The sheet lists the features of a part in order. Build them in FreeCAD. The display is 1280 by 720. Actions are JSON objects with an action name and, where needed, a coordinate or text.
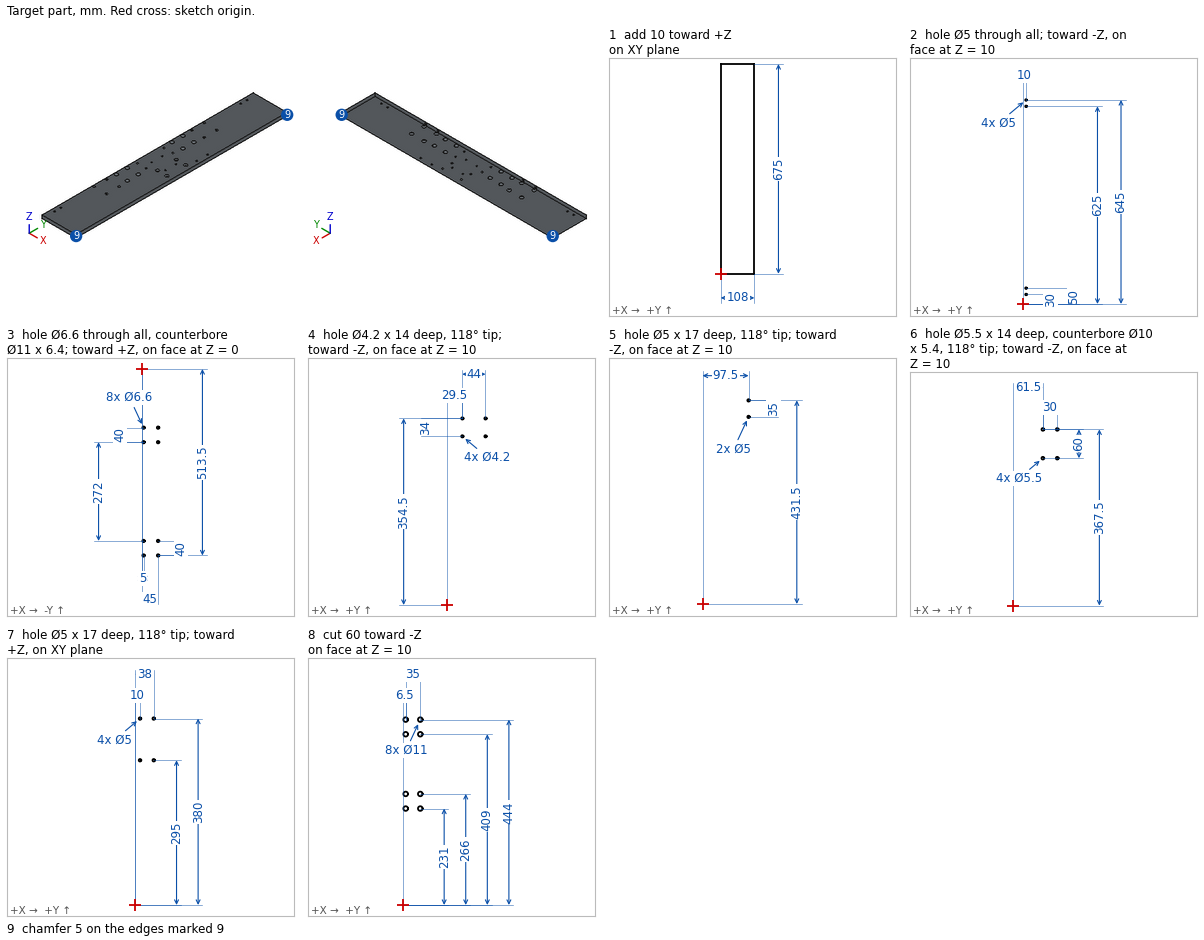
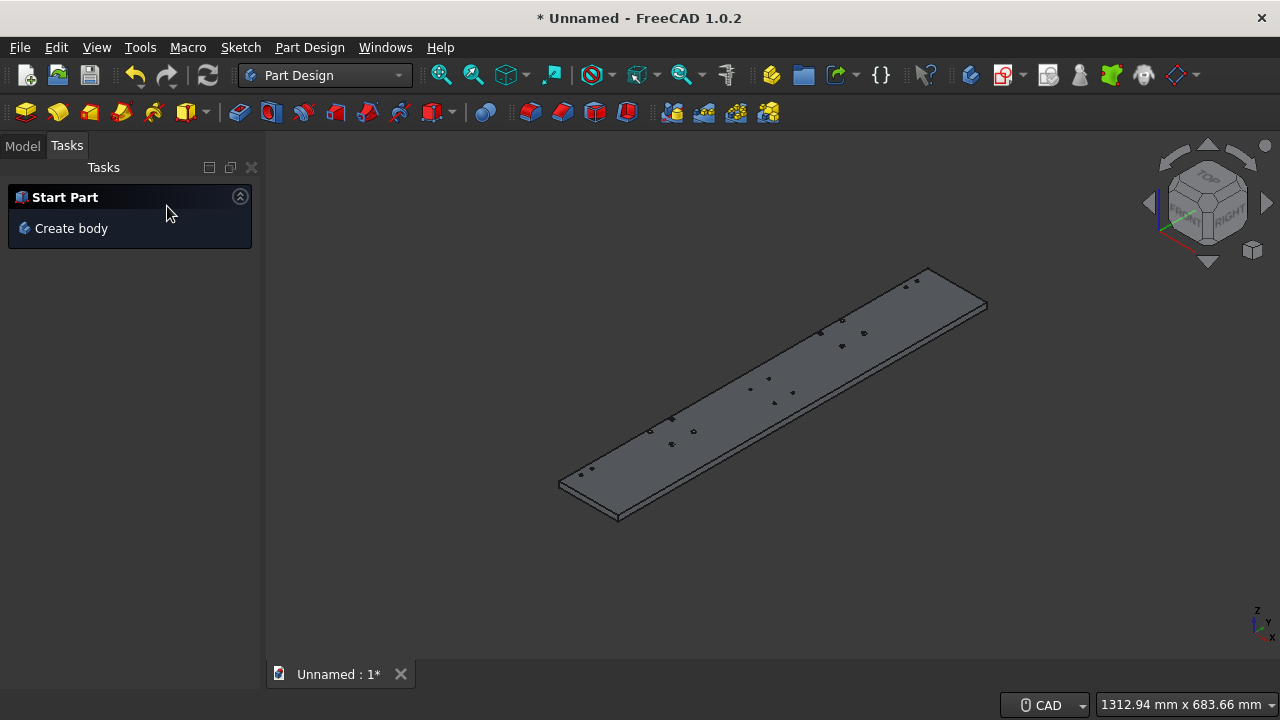
{"action": "left_click", "coordinate": [931, 300]}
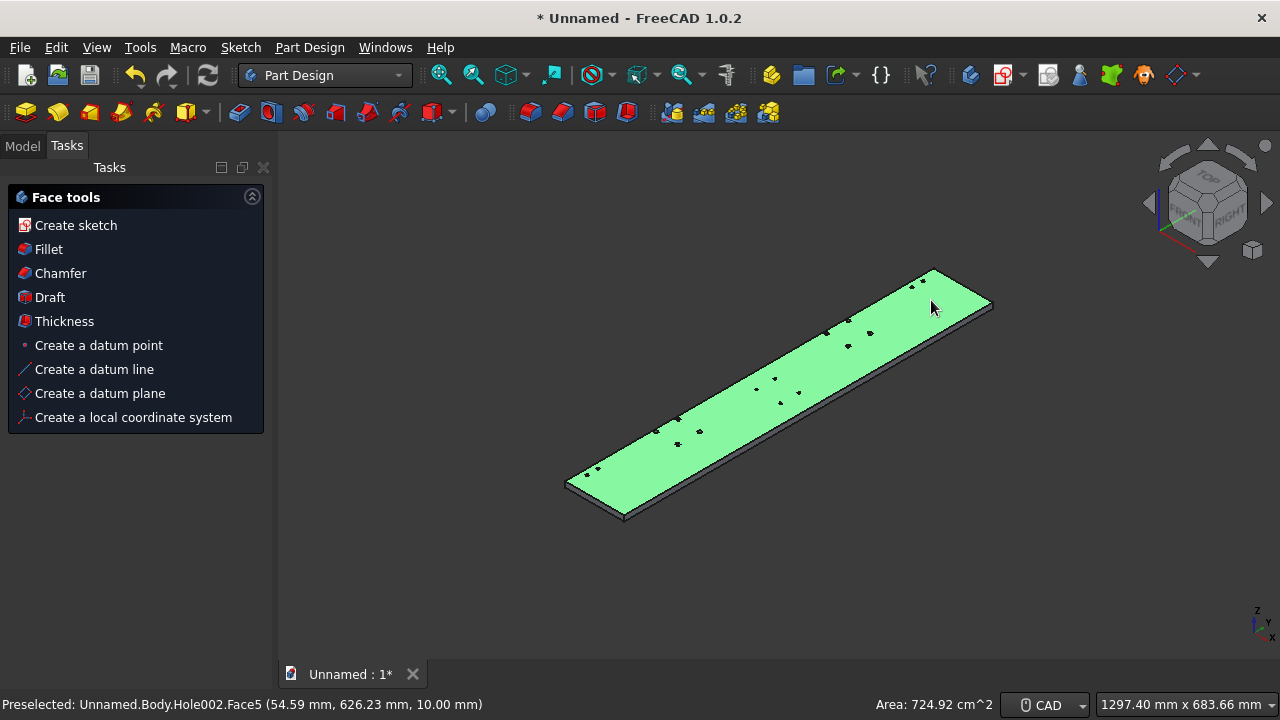
{"action": "left_click", "coordinate": [1004, 76]}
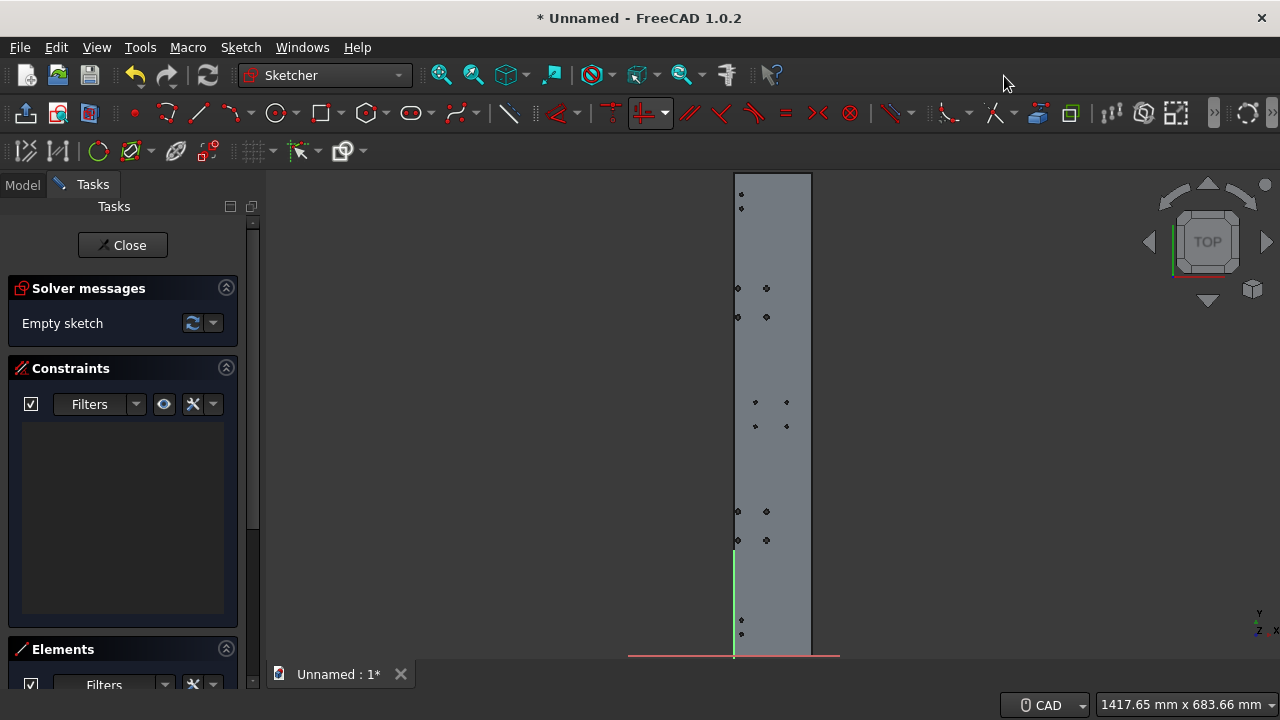
{"action": "scroll", "coordinate": [814, 354], "scroll_direction": "up", "scroll_amount": 12}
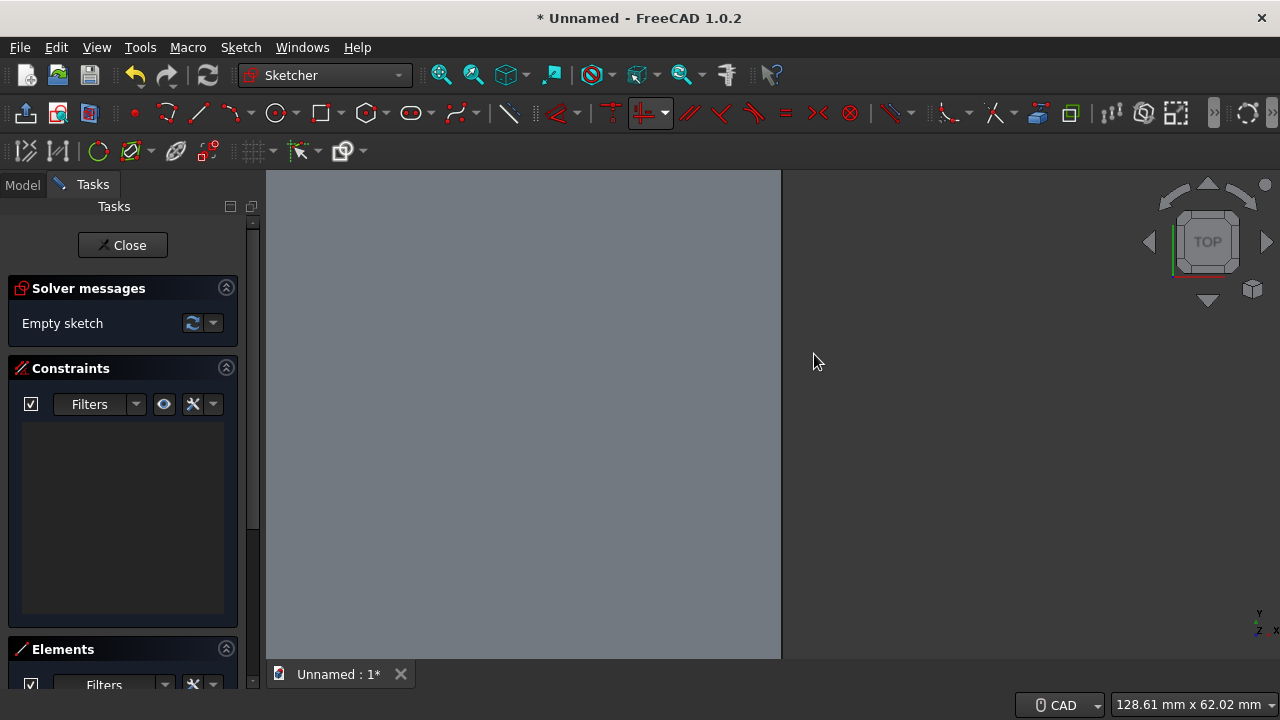
{"action": "left_click", "coordinate": [276, 114]}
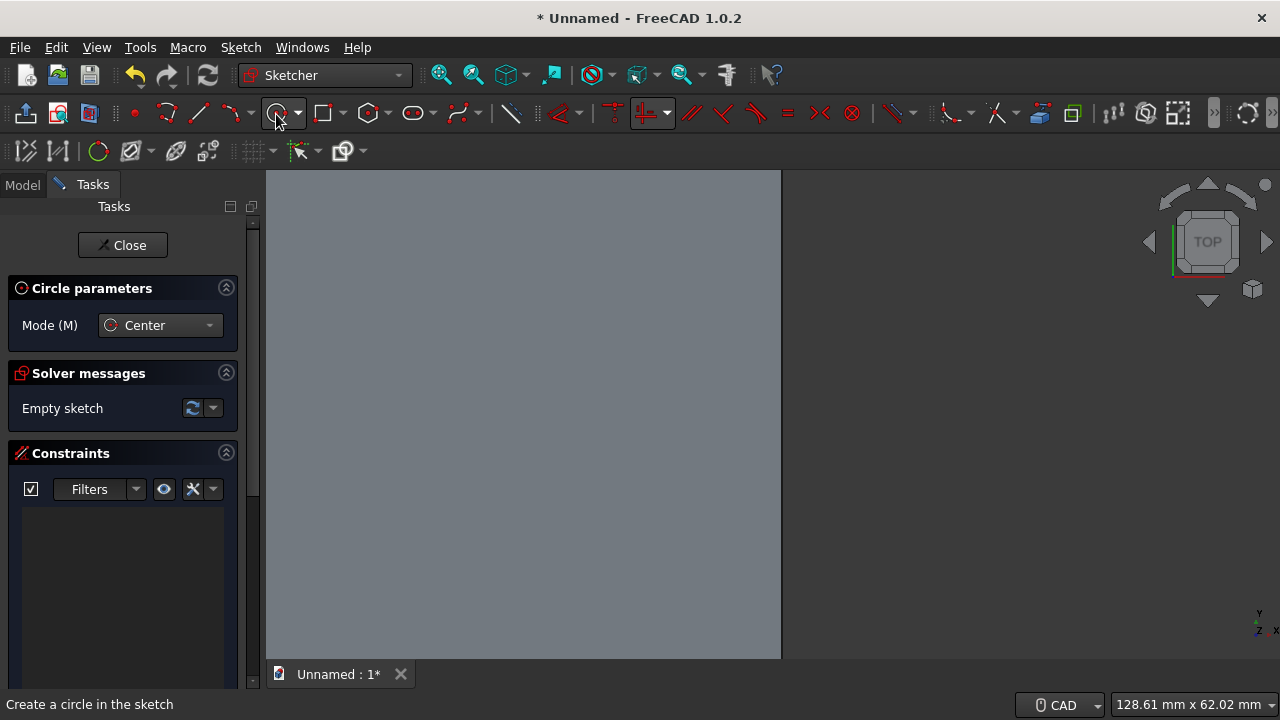
{"action": "left_click", "coordinate": [700, 276]}
{"action": "mouse_move", "coordinate": [714, 262]}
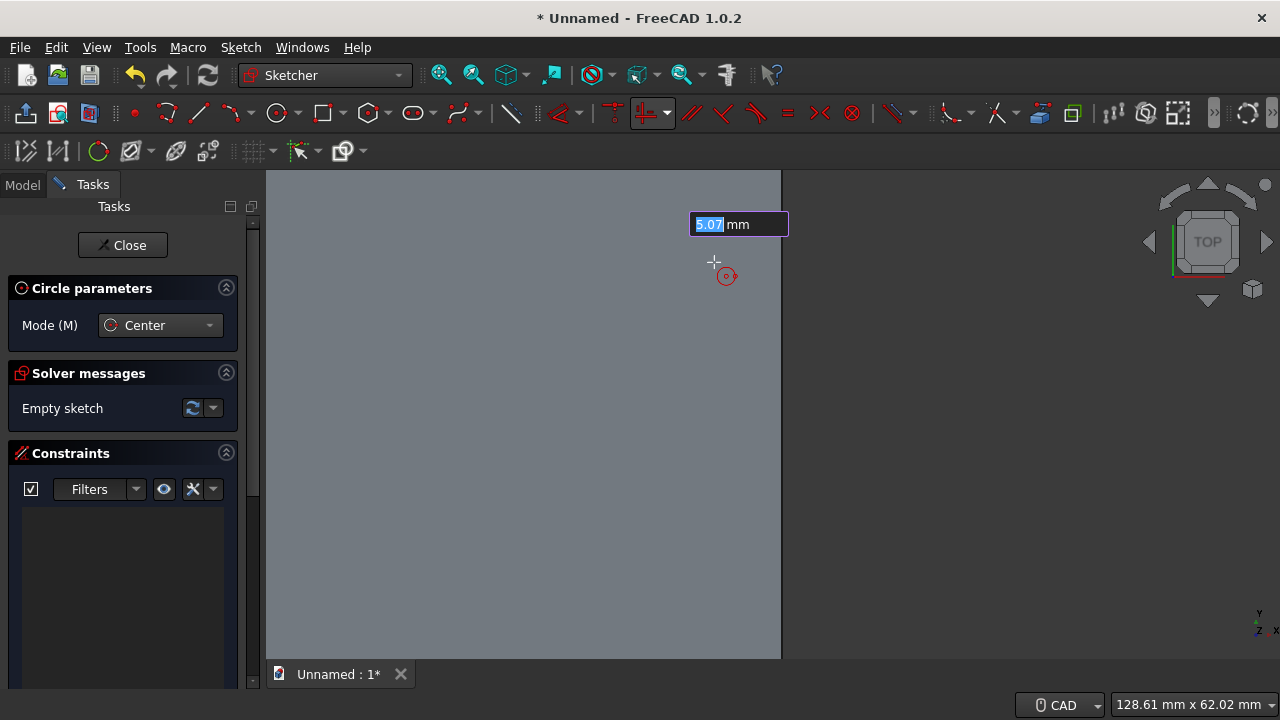
{"action": "type", "text": "5"}
{"action": "key", "text": "Return"}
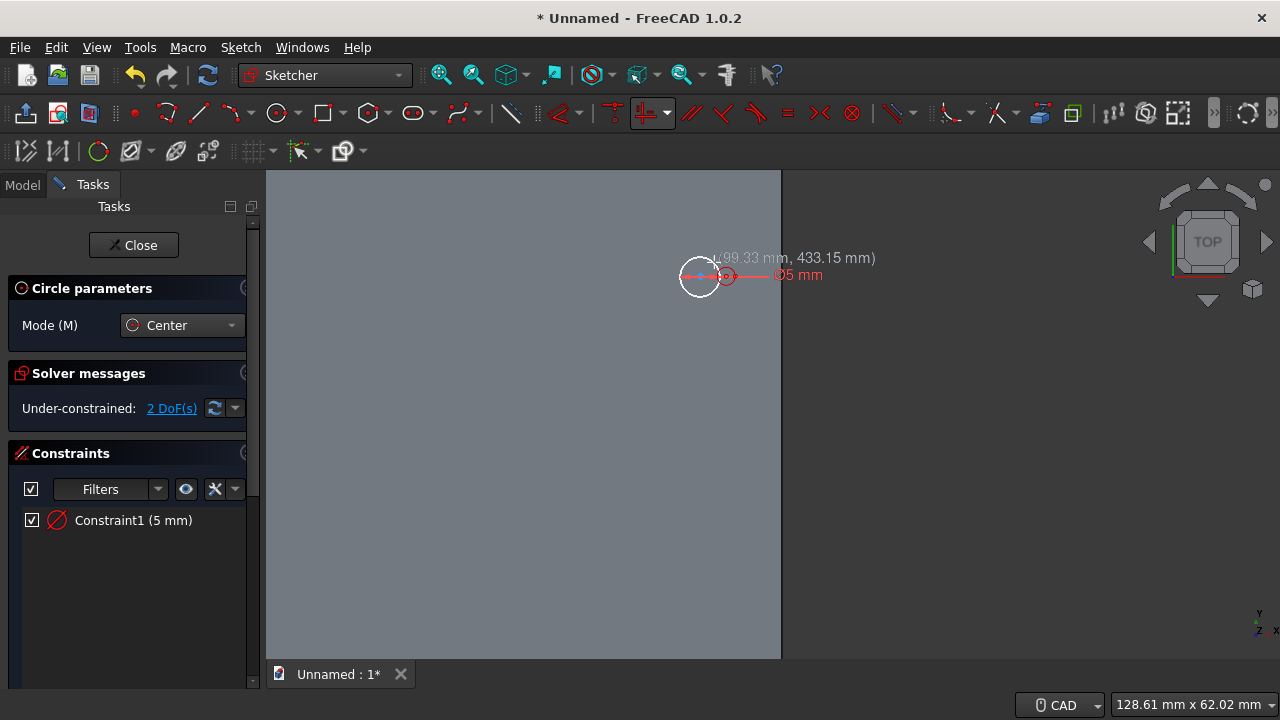
{"action": "left_click", "coordinate": [700, 552]}
{"action": "mouse_move", "coordinate": [714, 538]}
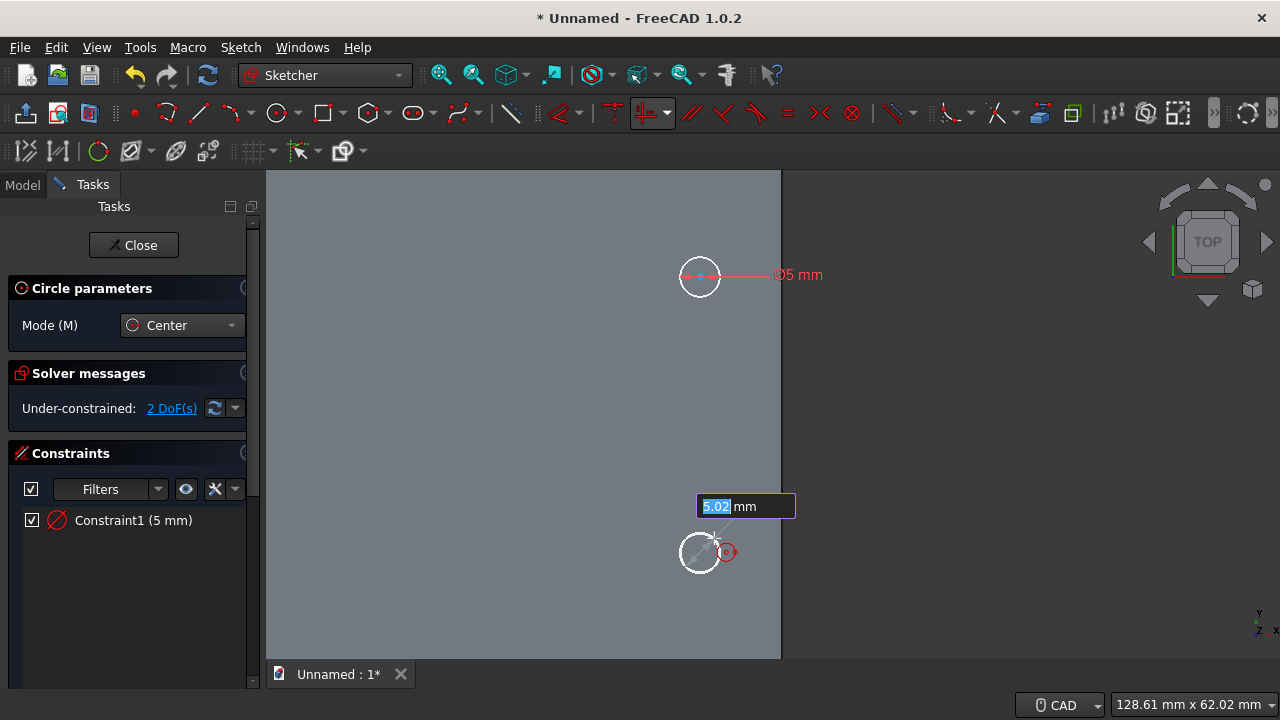
{"action": "type", "text": "5"}
{"action": "key", "text": "Return"}
{"action": "key", "text": "Escape"}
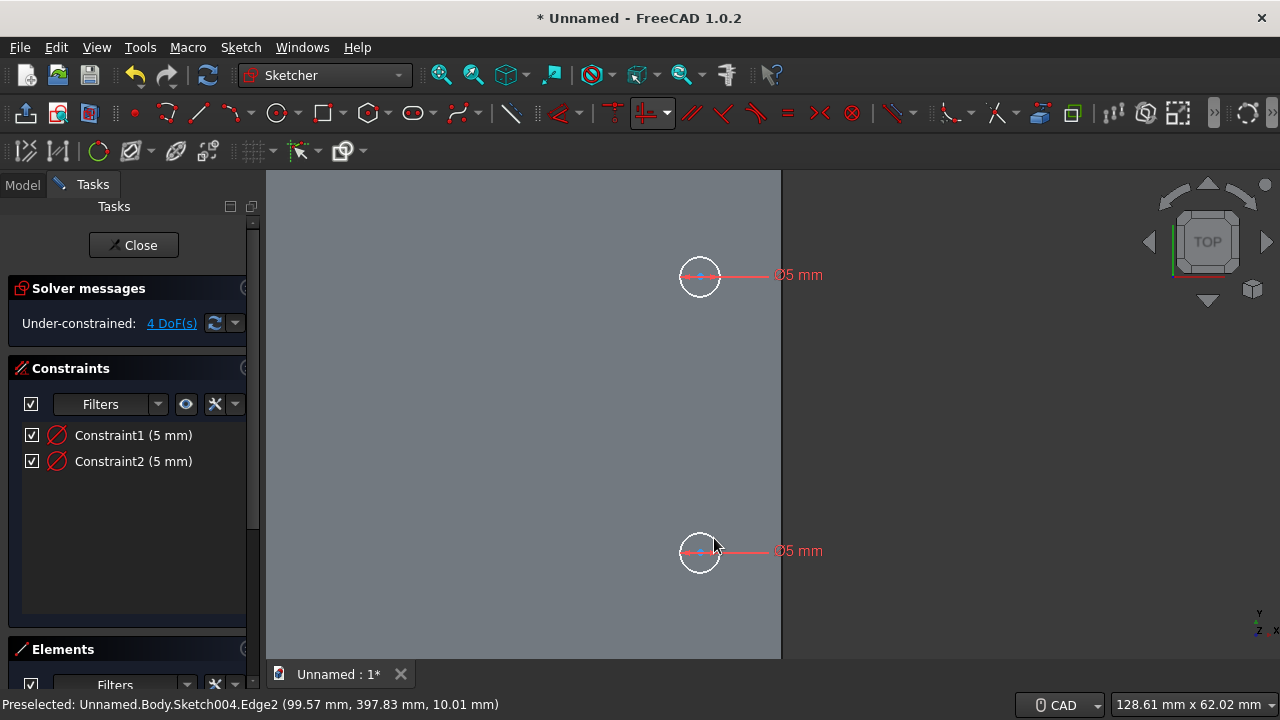
{"action": "left_click", "coordinate": [700, 277]}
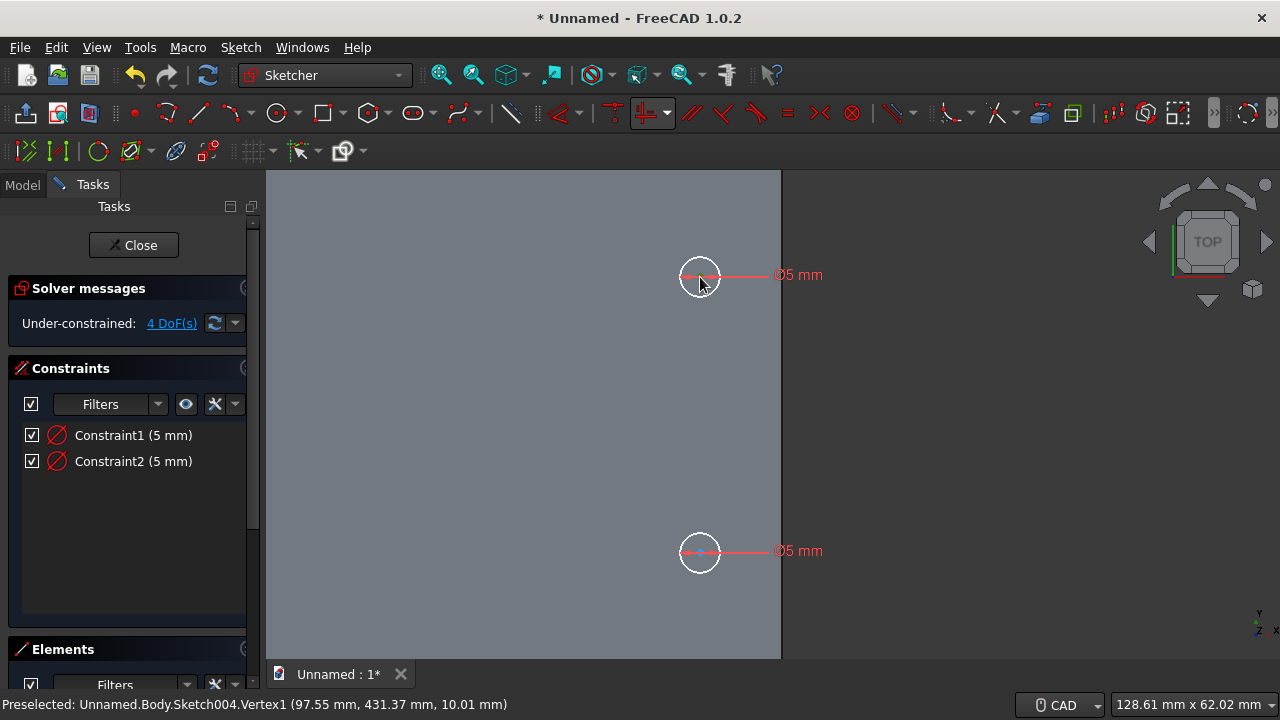
{"action": "left_click", "coordinate": [700, 553]}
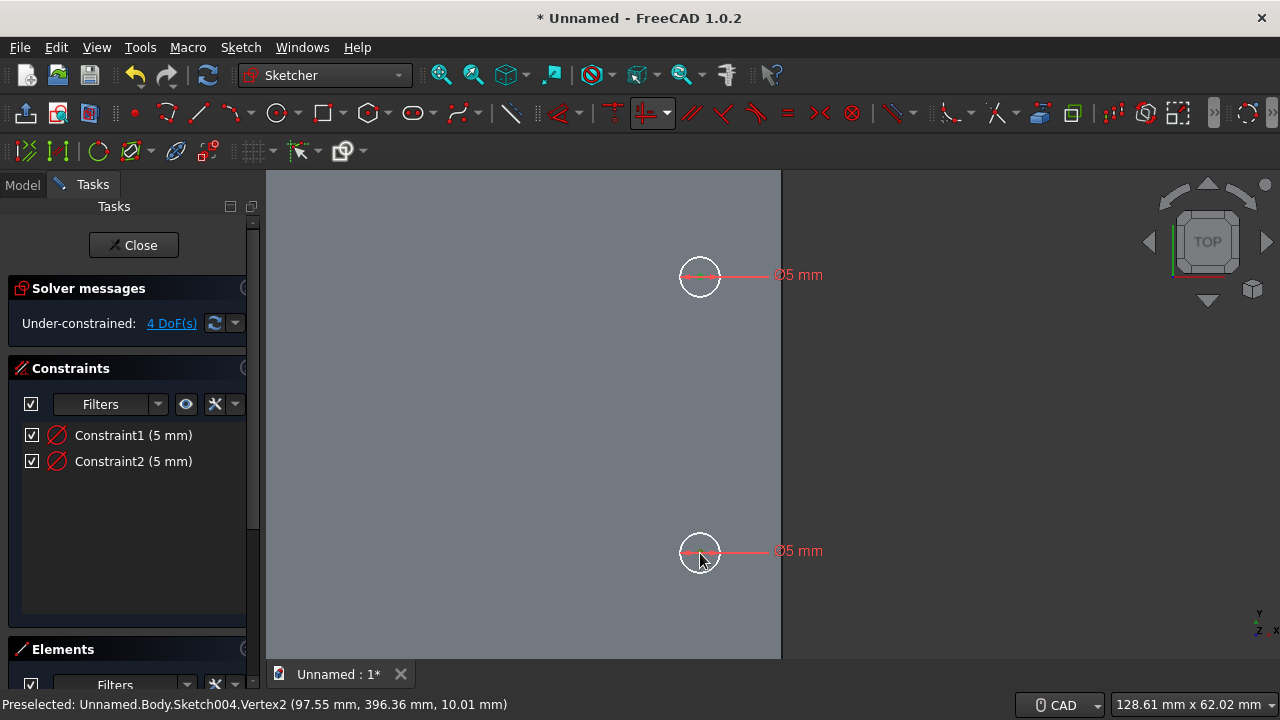
{"action": "key", "text": "v"}